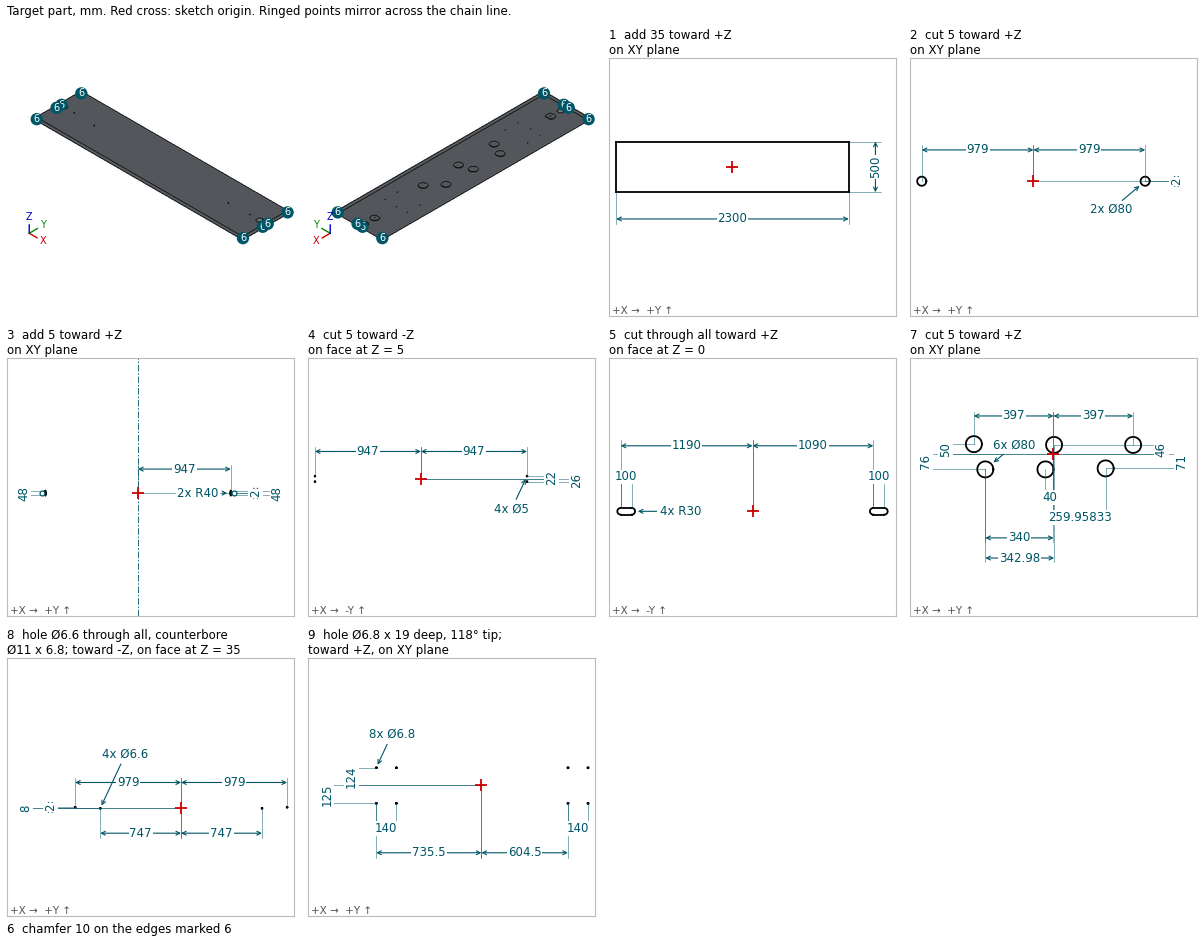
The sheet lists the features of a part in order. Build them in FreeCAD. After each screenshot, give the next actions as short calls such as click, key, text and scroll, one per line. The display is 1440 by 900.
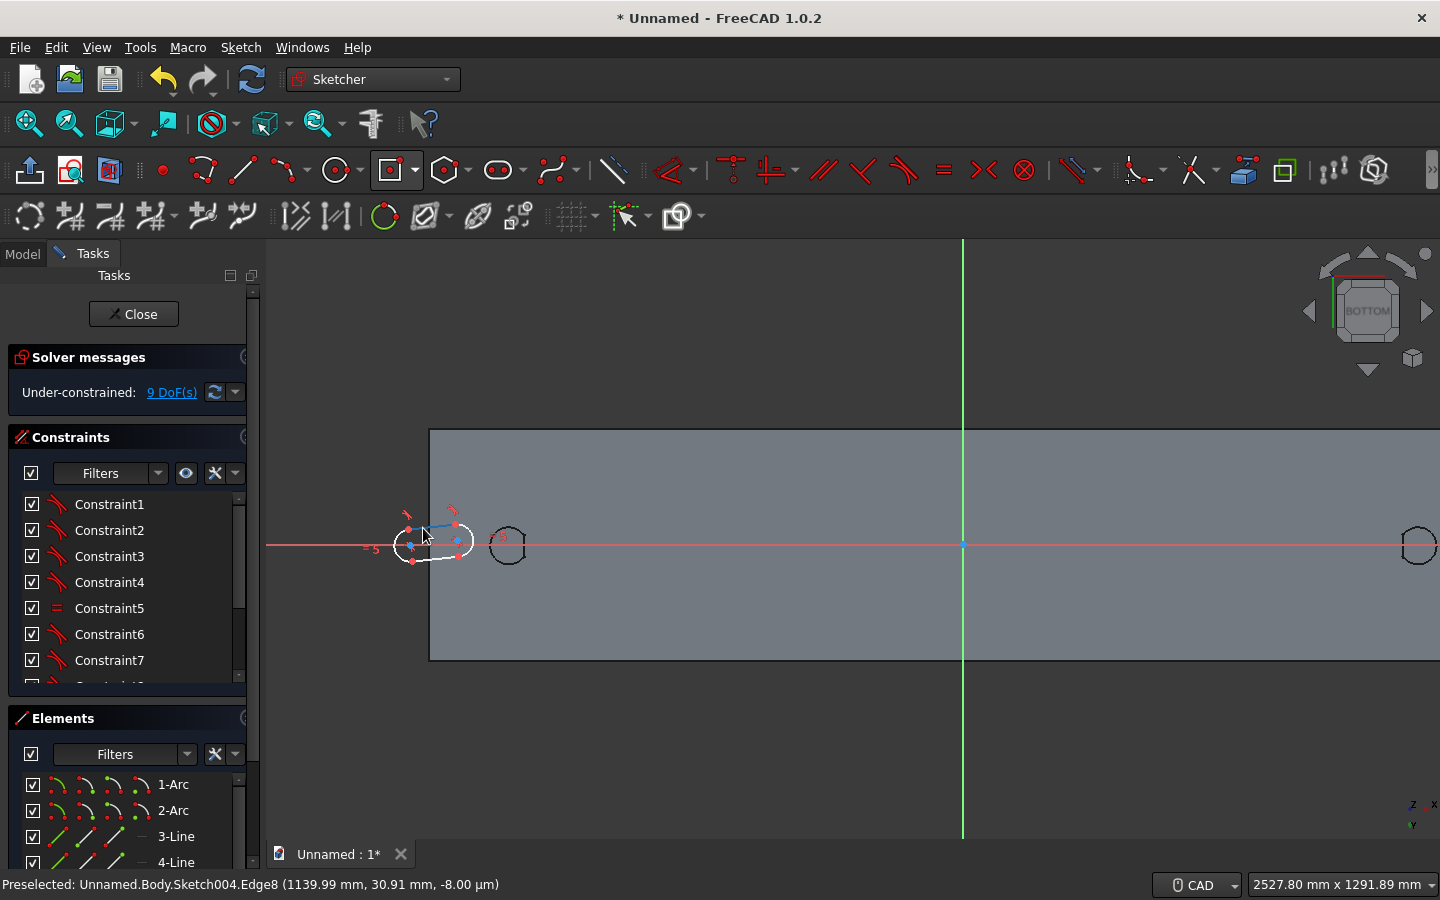
click(423, 528)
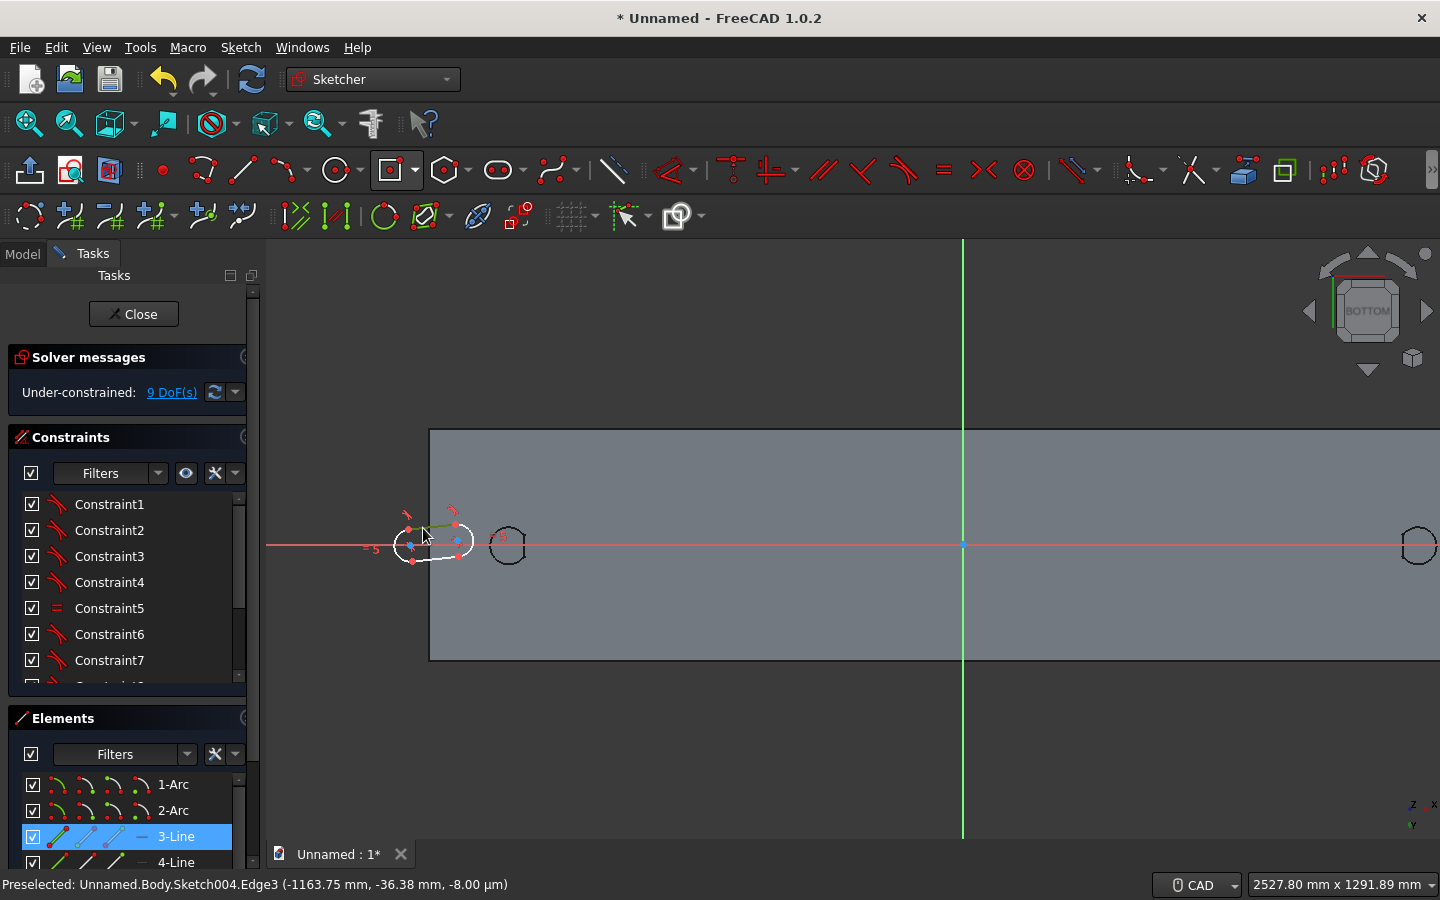
click(798, 170)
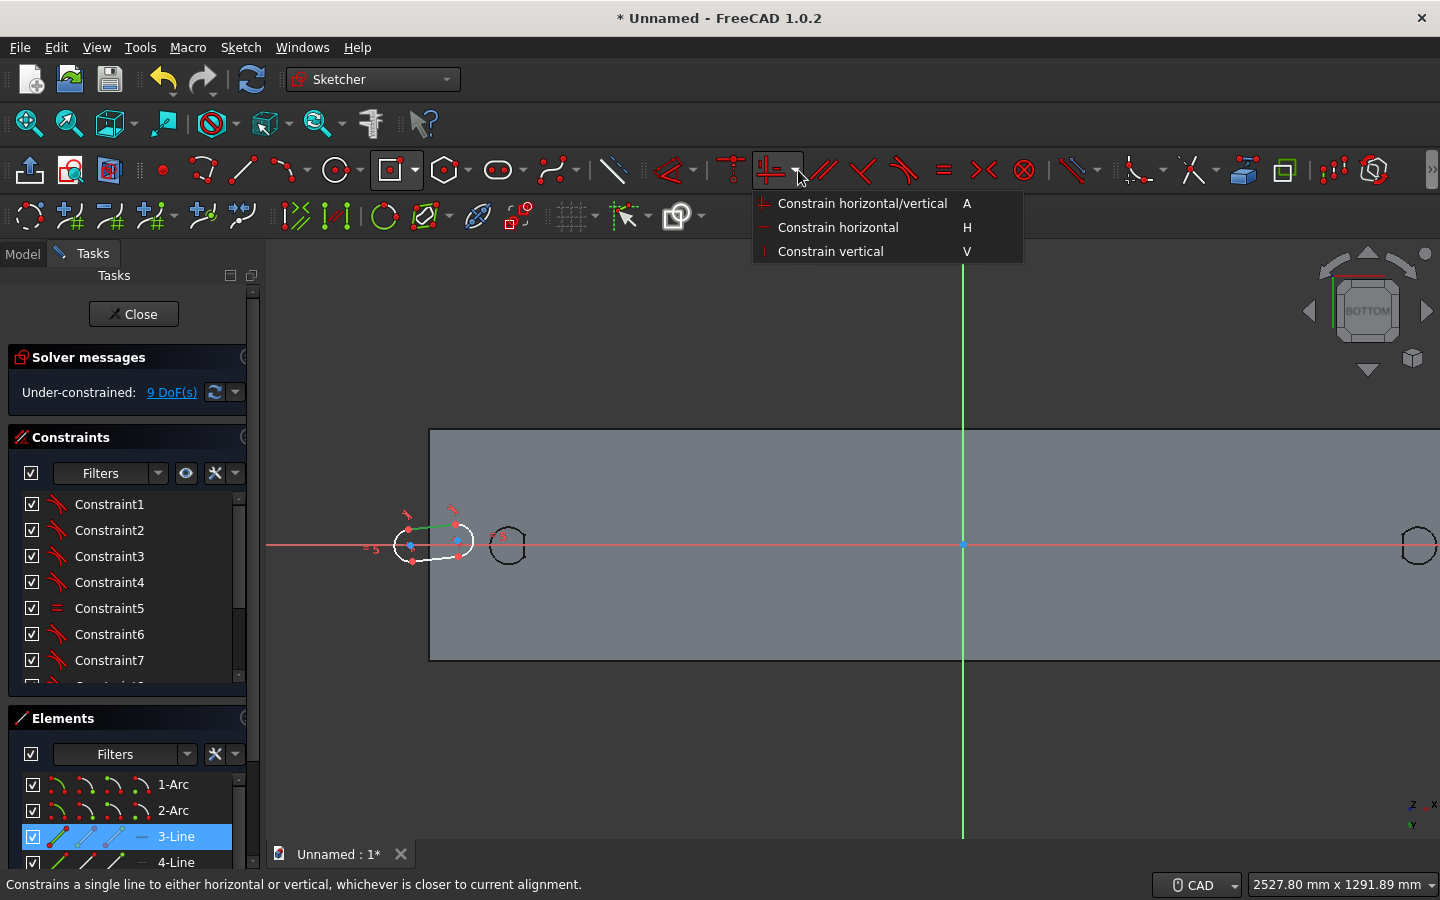
click(888, 227)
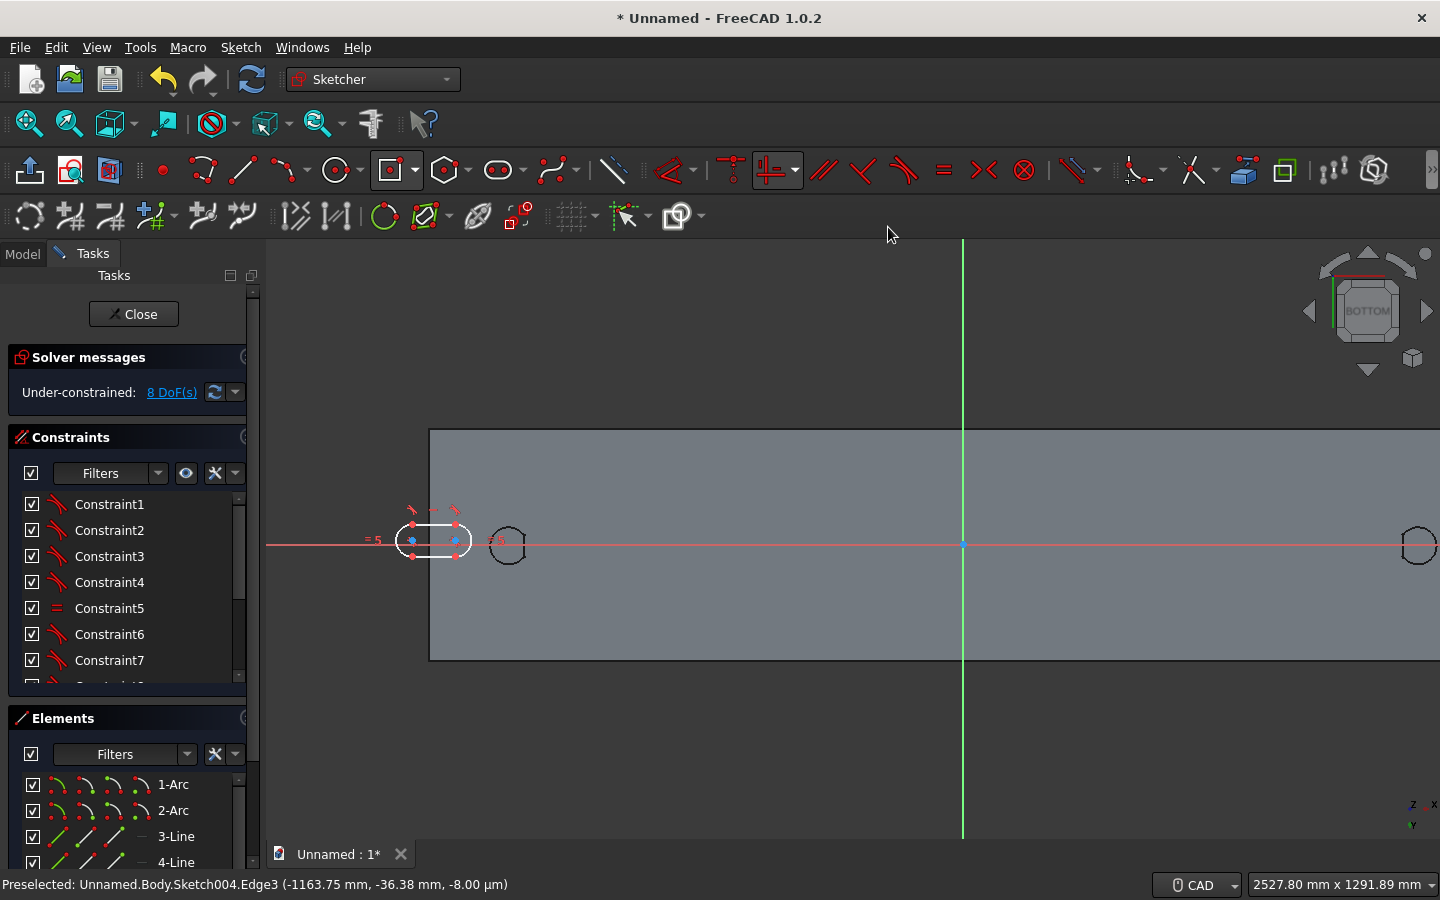
scroll(421, 527, down, 2)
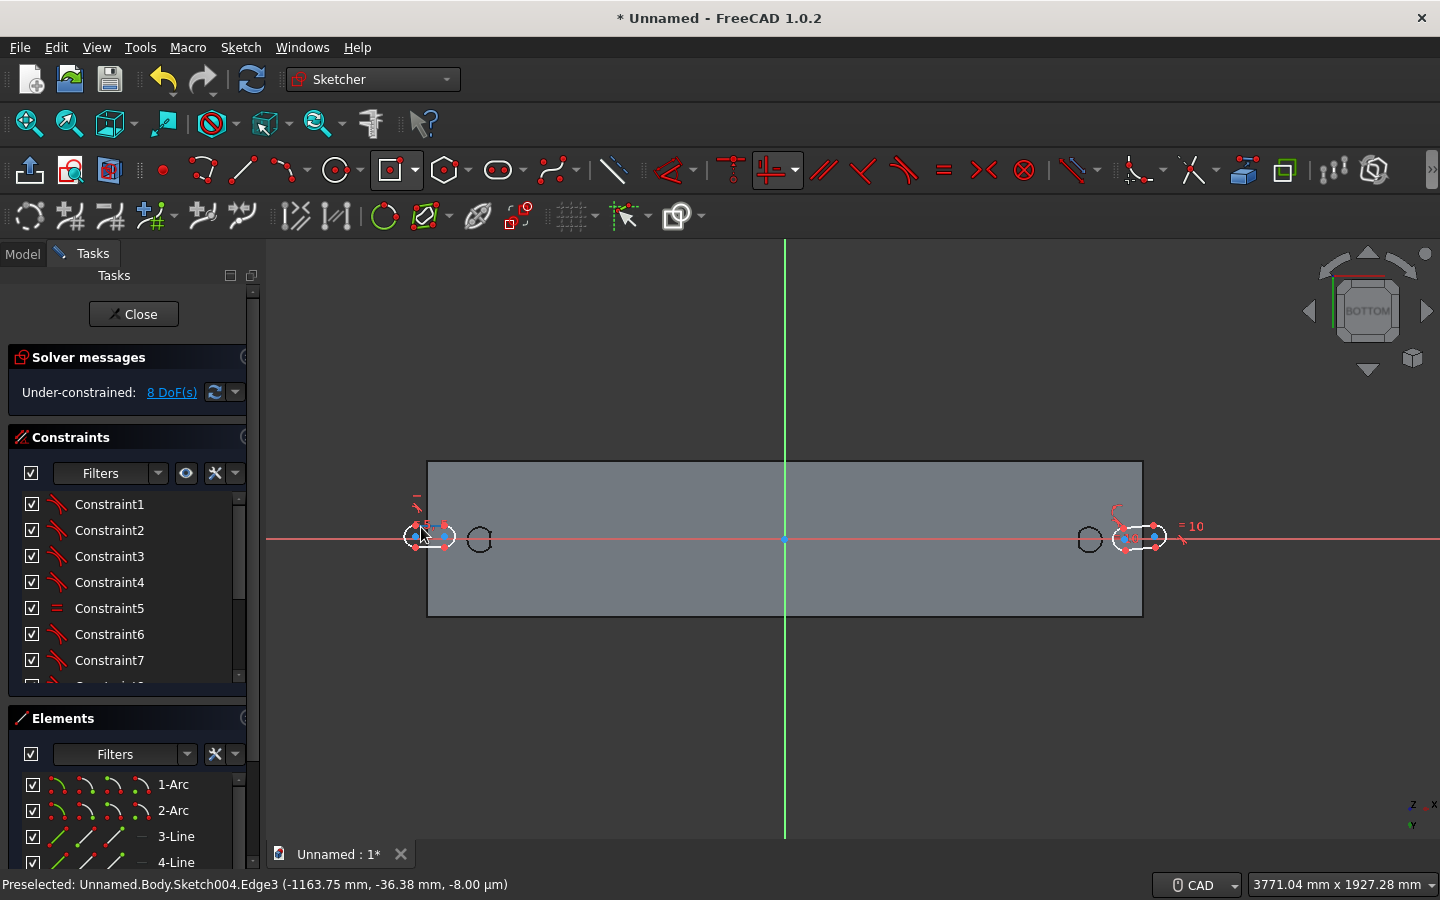
scroll(1132, 527, up, 2)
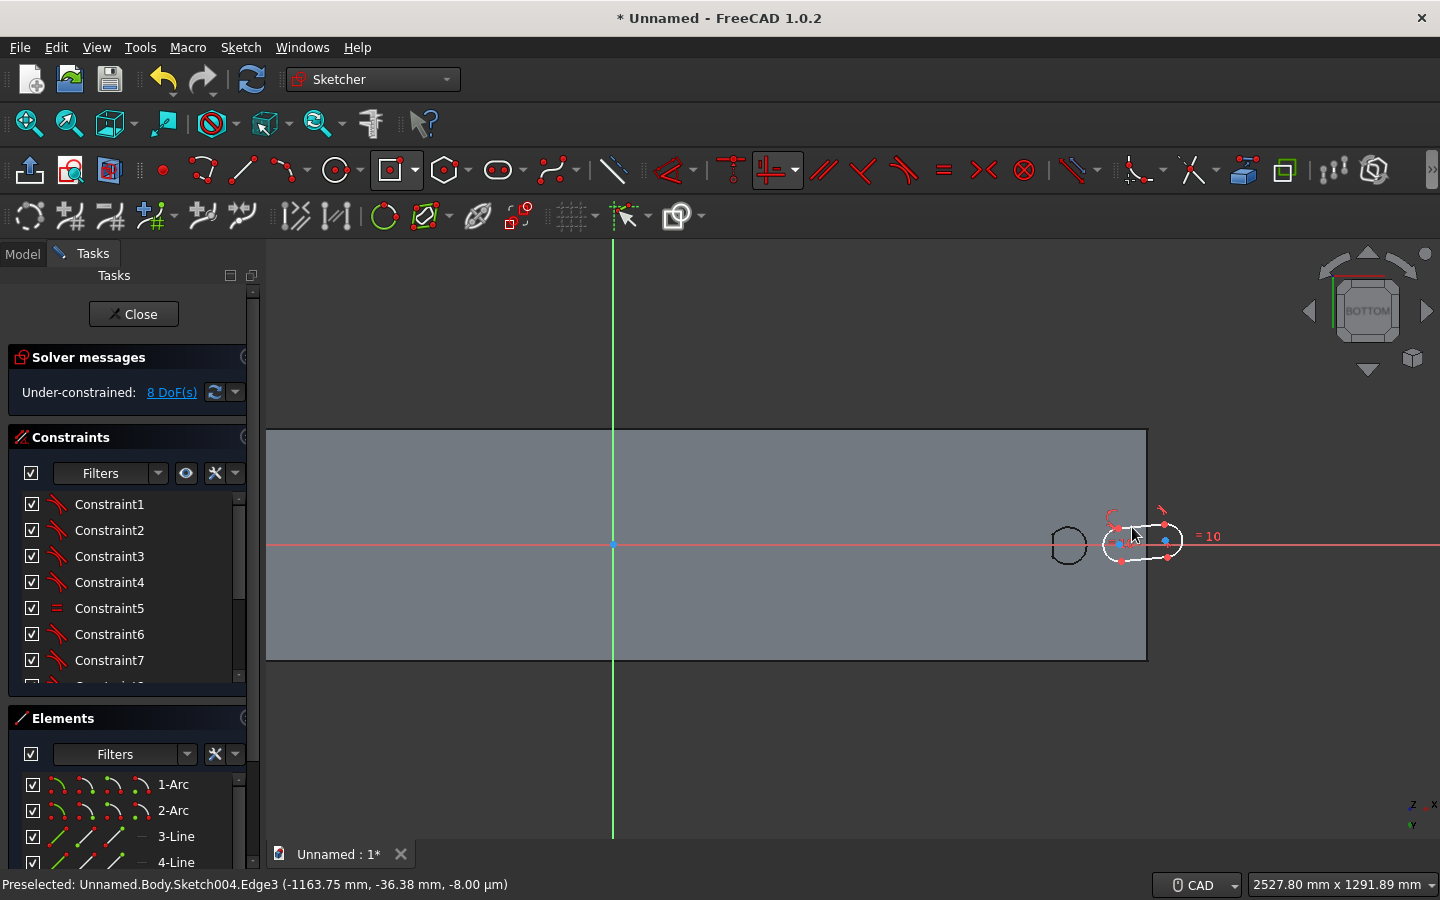
click(1151, 526)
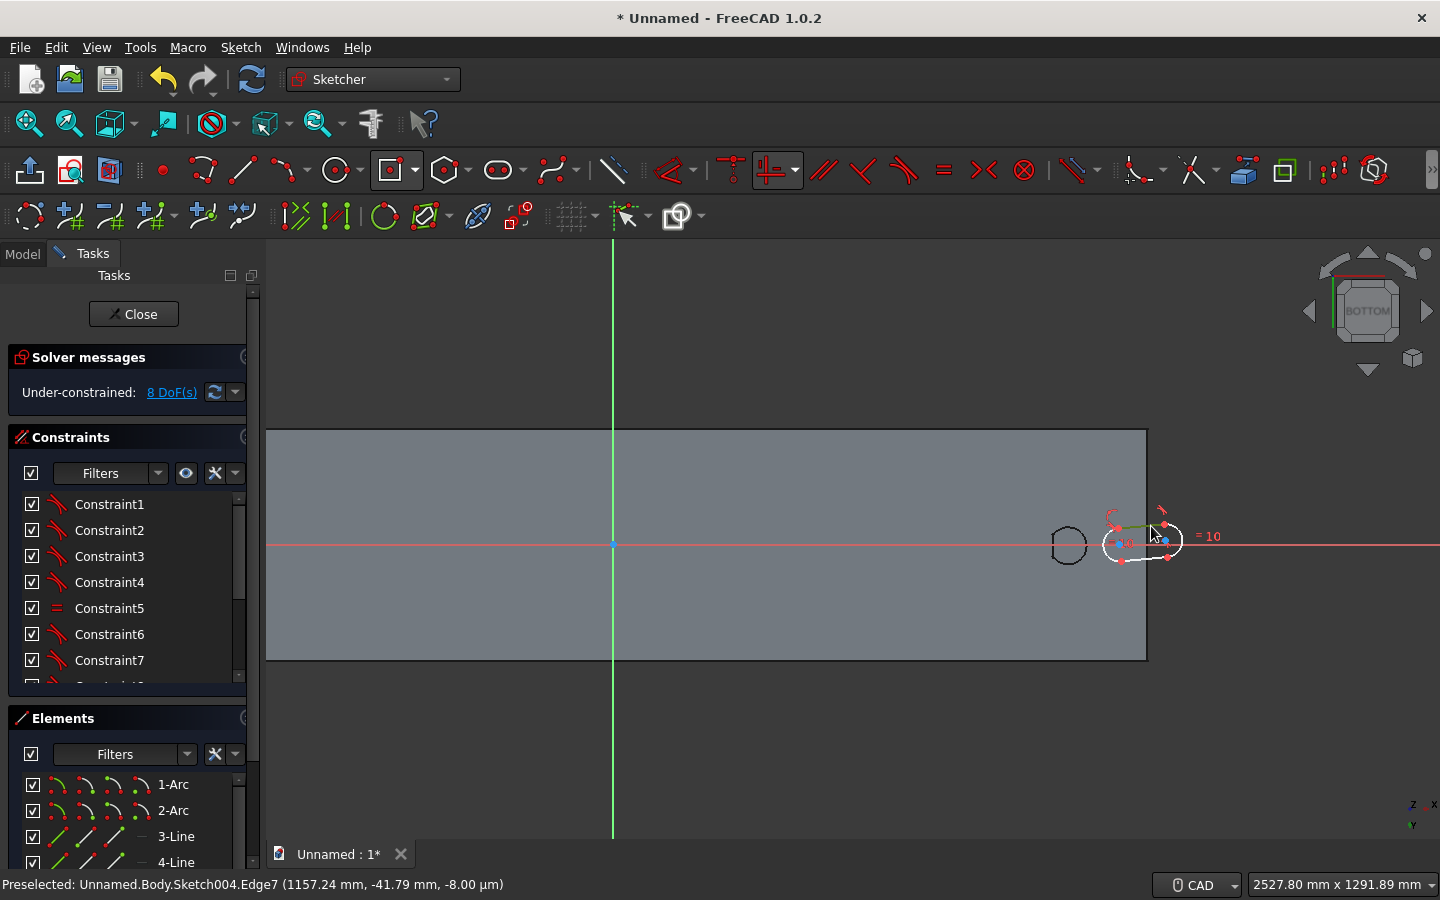
click(798, 170)